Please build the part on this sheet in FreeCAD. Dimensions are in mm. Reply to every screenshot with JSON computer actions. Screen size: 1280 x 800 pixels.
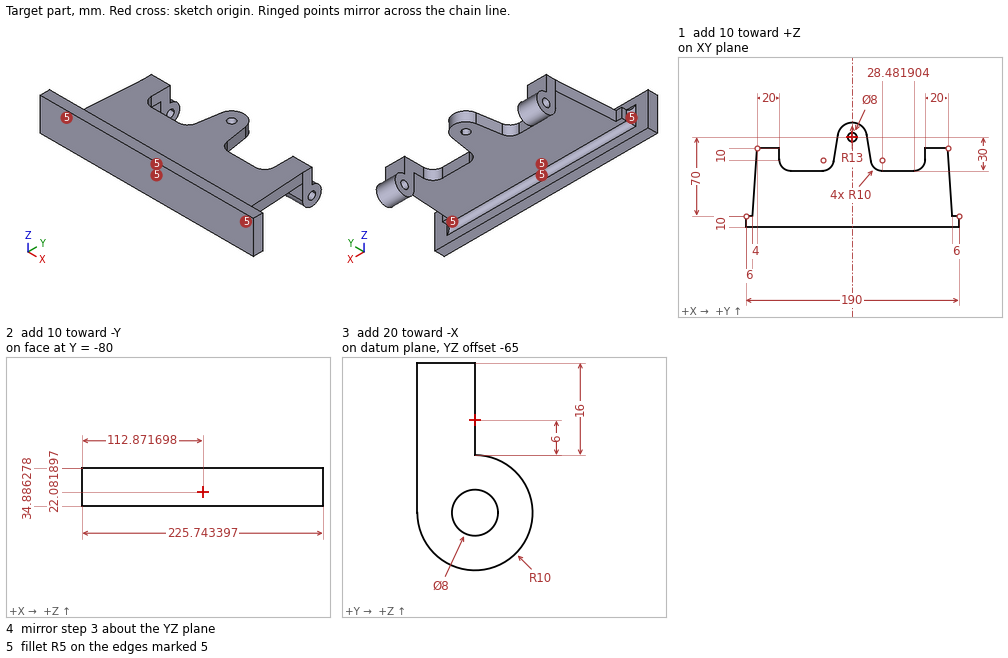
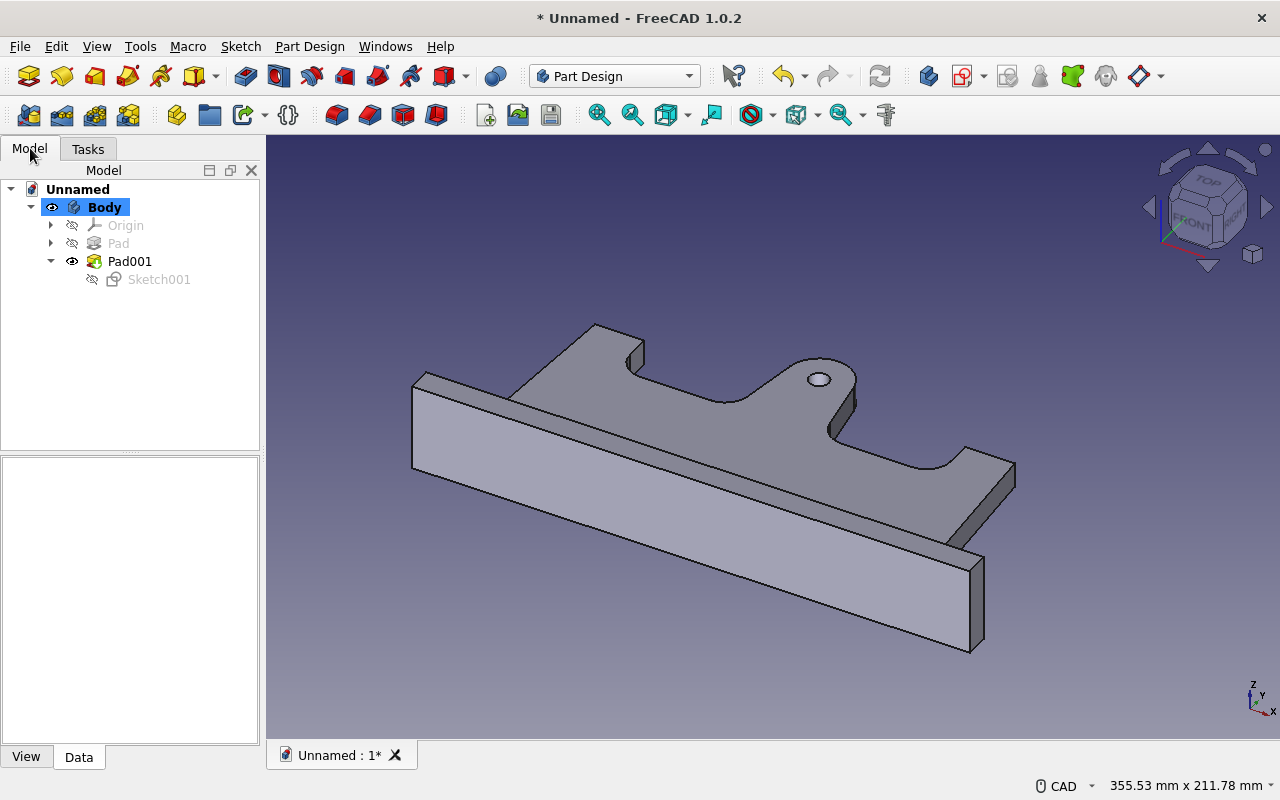
{"action": "left_click", "coordinate": [51, 225]}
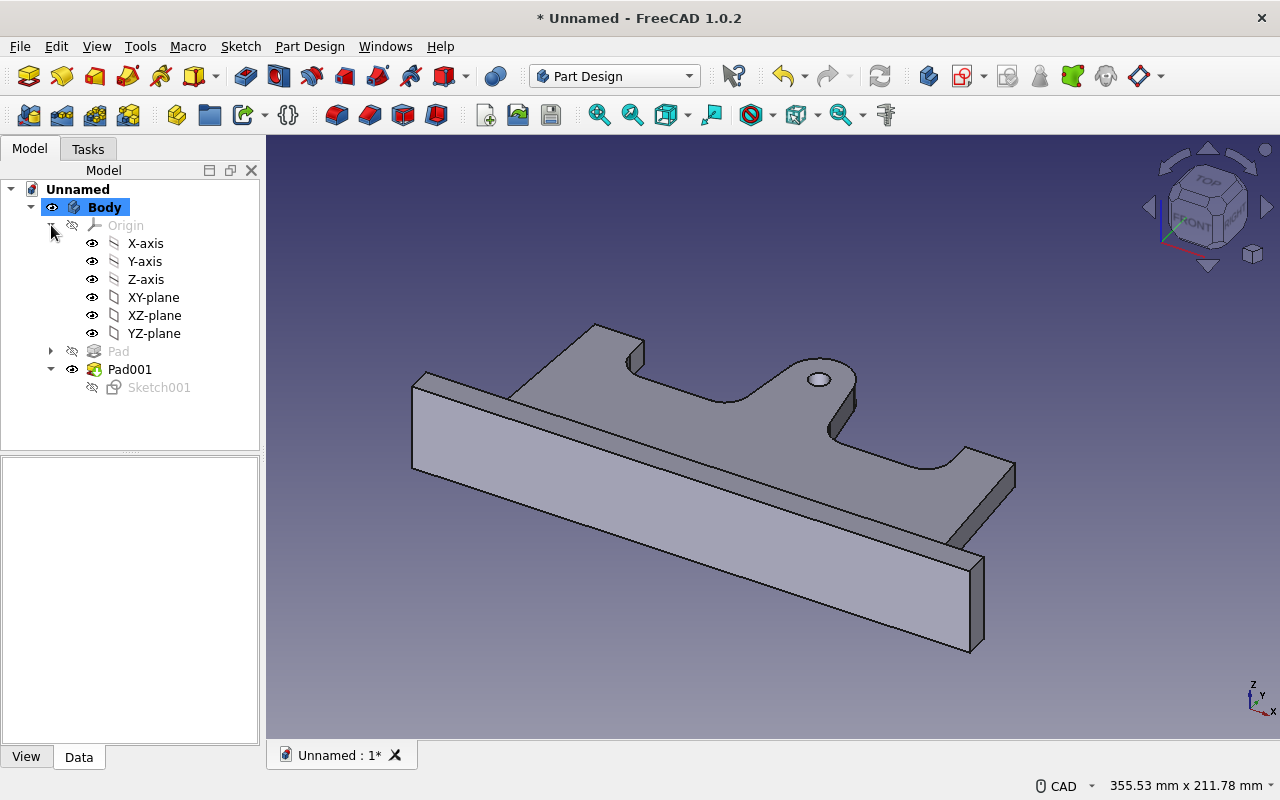
{"action": "left_click", "coordinate": [137, 333]}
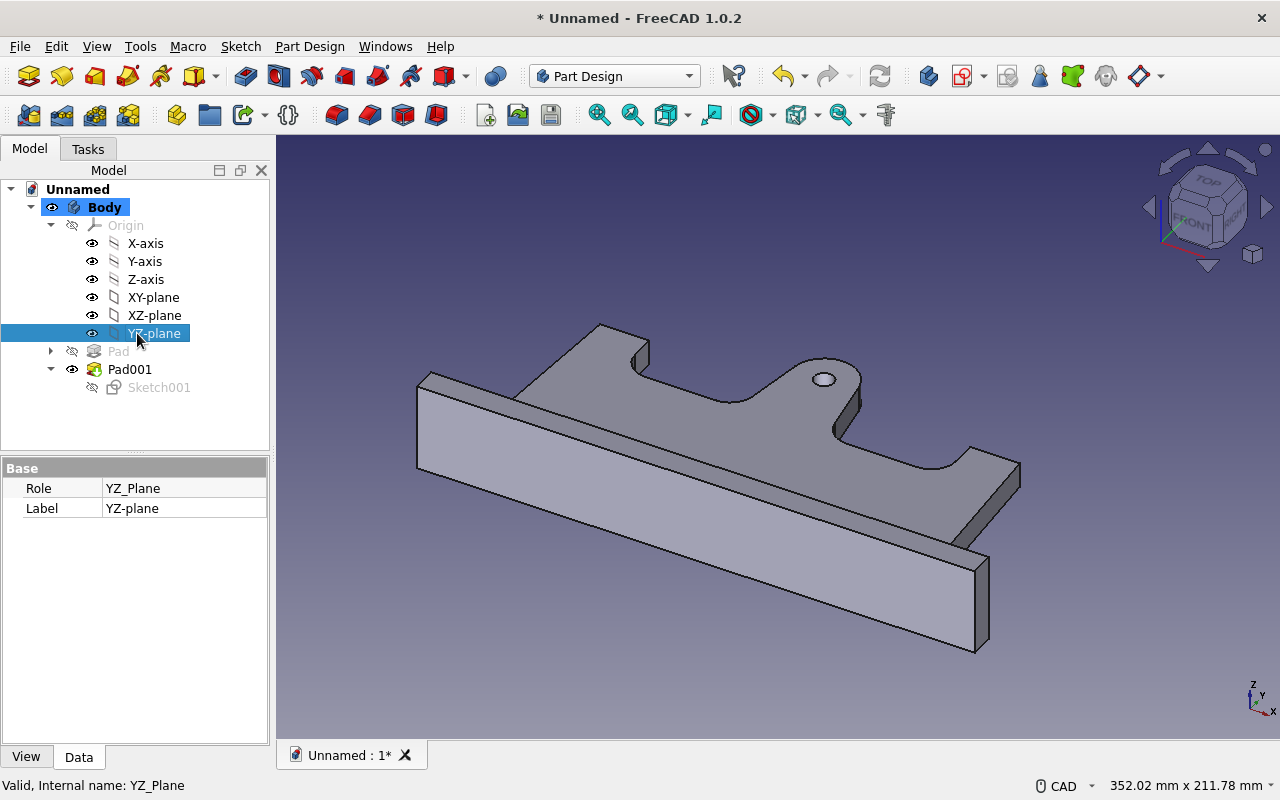
{"action": "left_click", "coordinate": [1138, 76]}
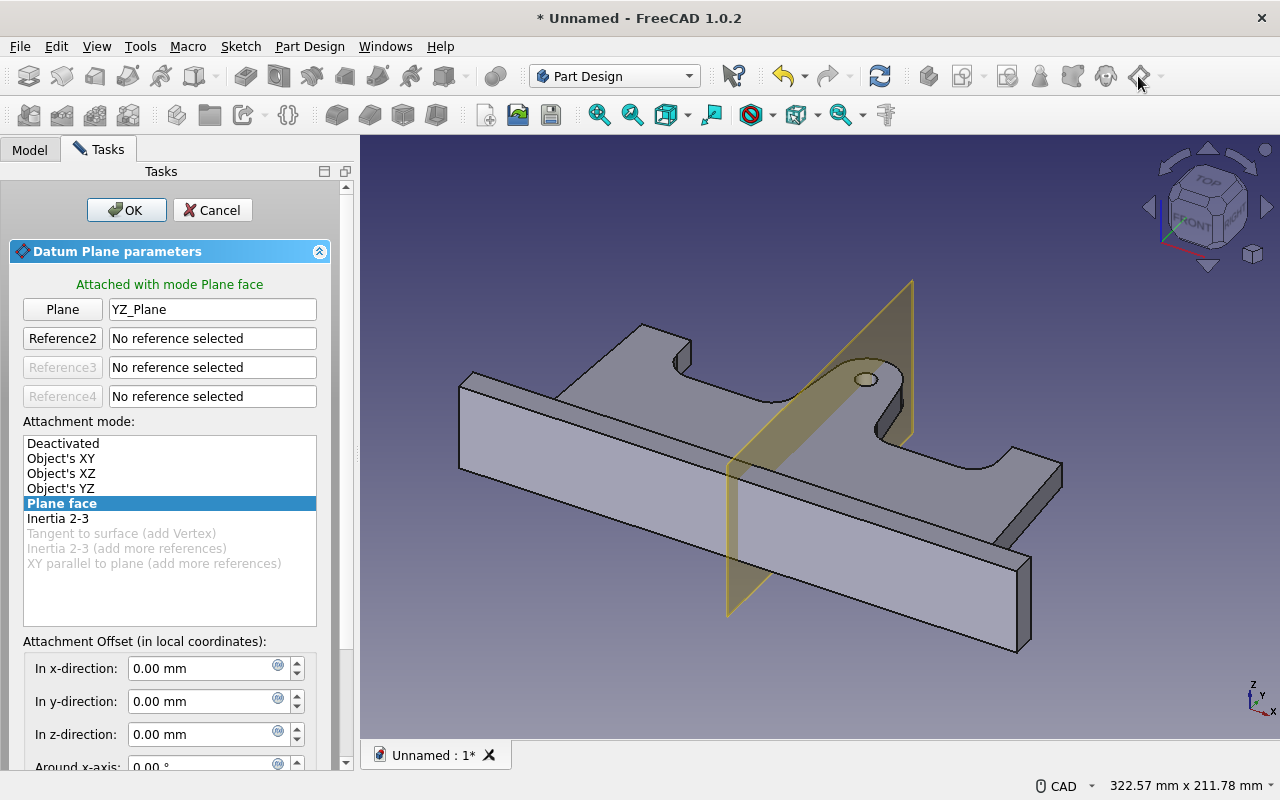
{"action": "triple_click", "coordinate": [210, 734]}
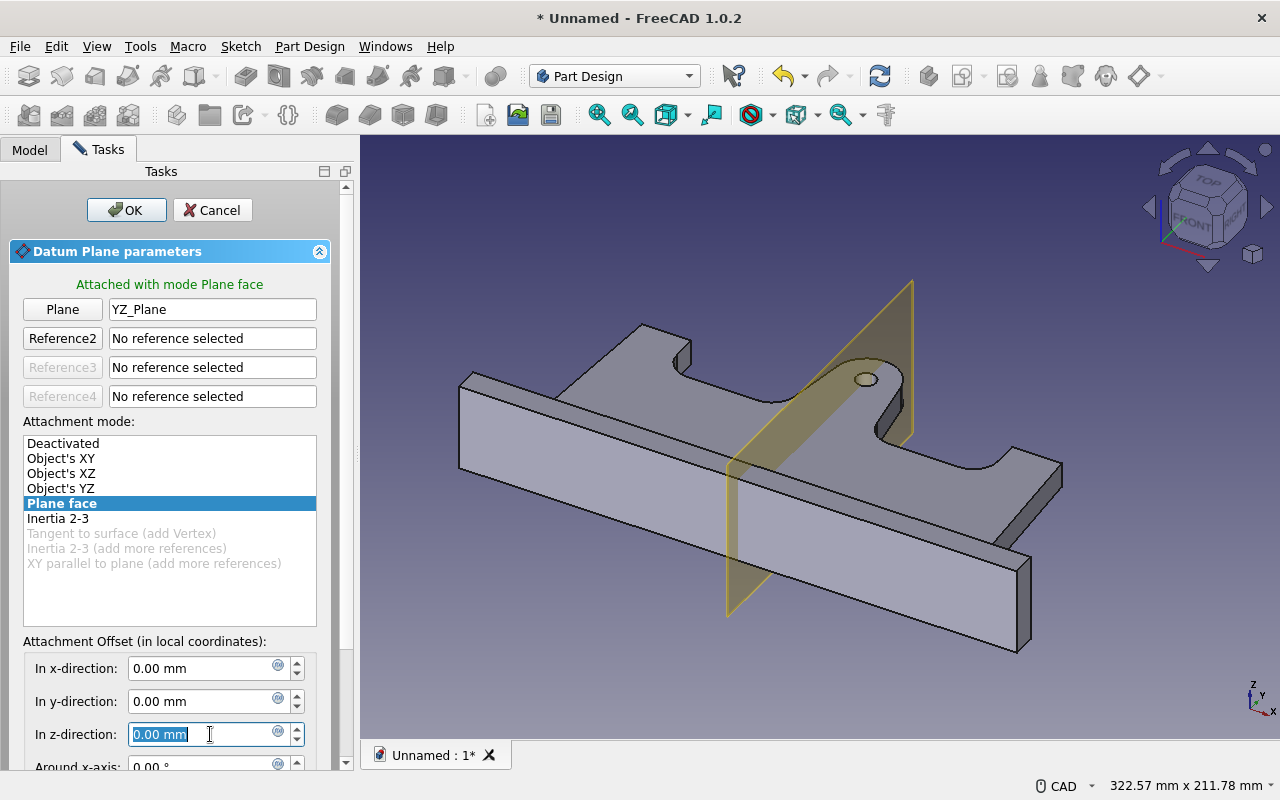
{"action": "type", "text": "-65"}
{"action": "key", "text": "Tab"}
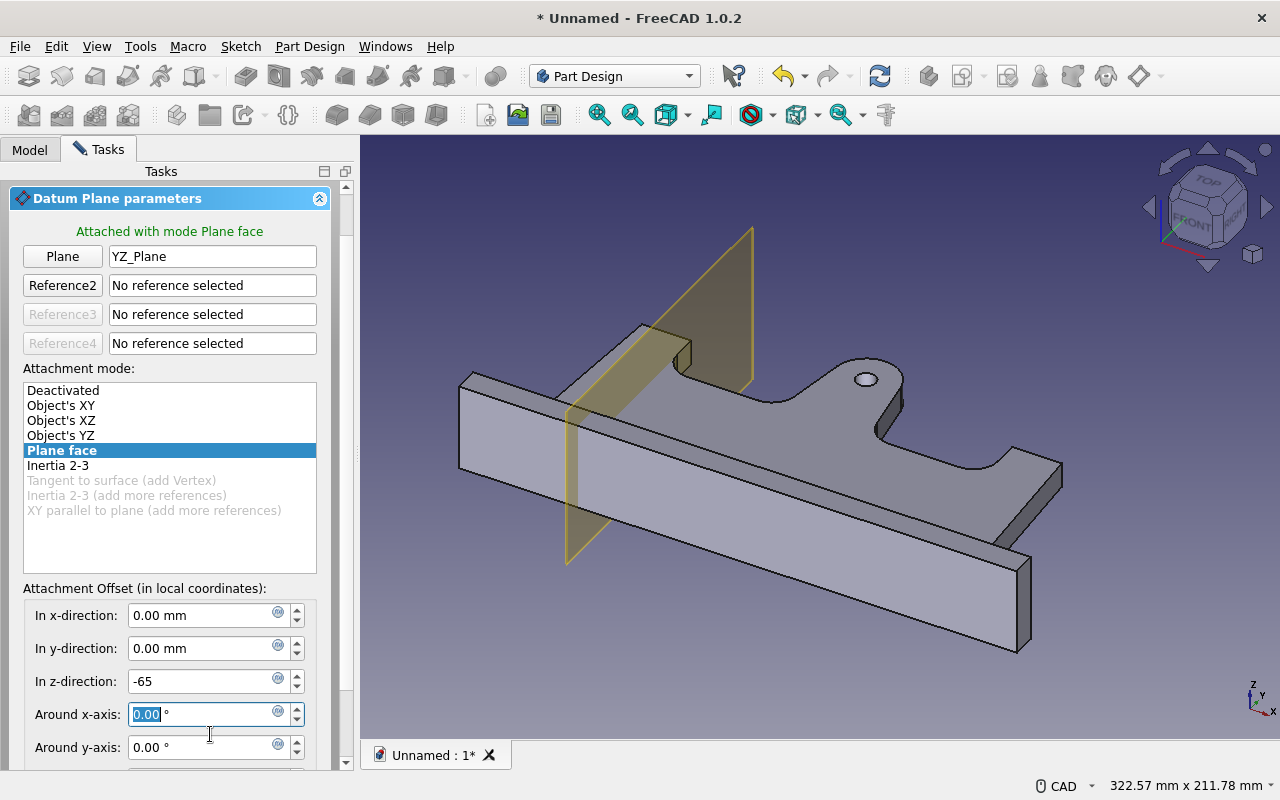
{"action": "scroll", "coordinate": [346, 476], "scroll_direction": "up", "scroll_amount": 2}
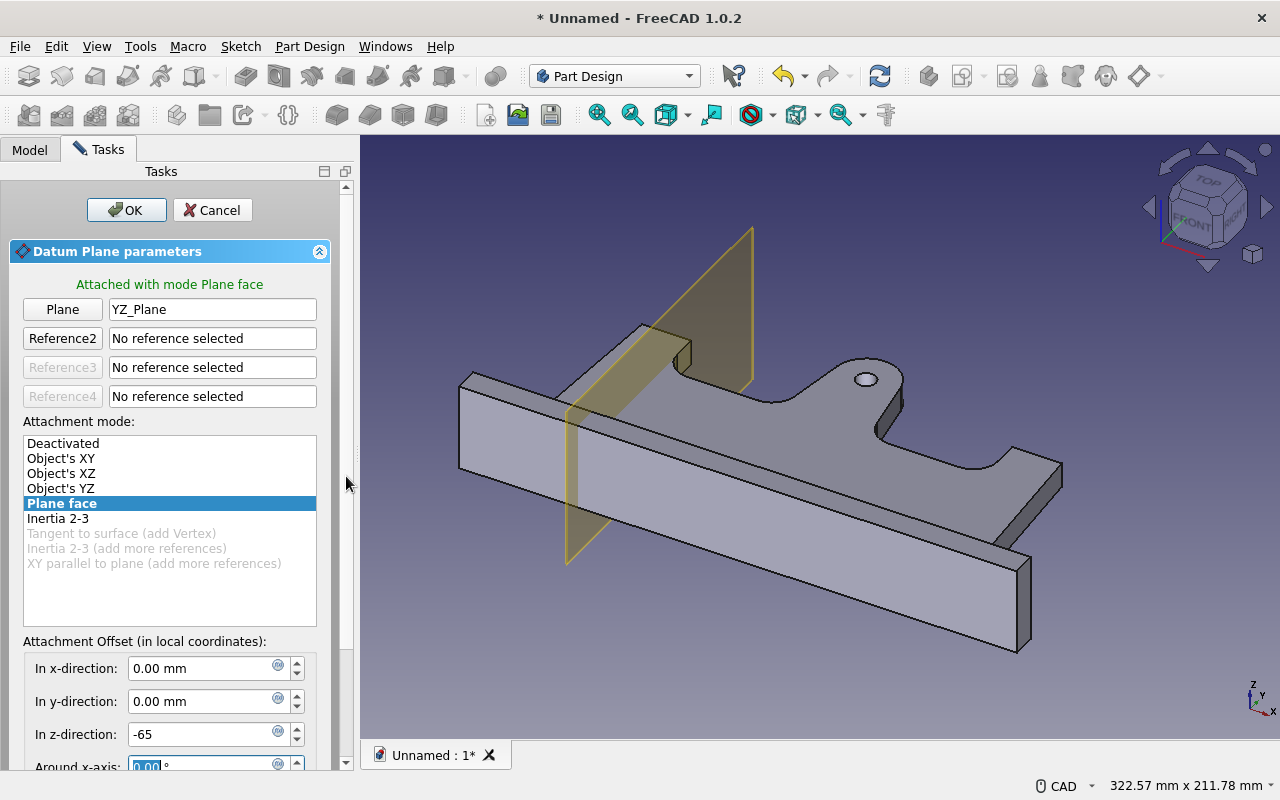
{"action": "left_click", "coordinate": [127, 210]}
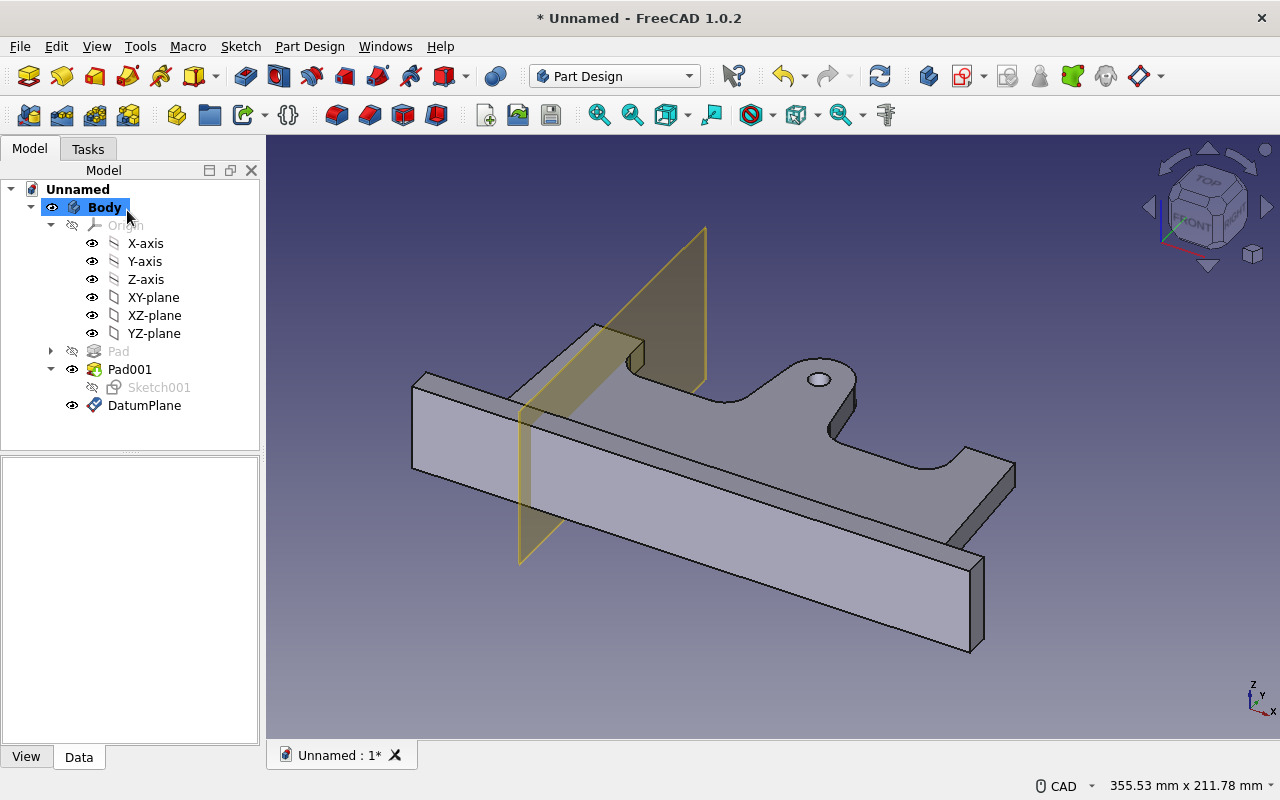
{"action": "left_click", "coordinate": [117, 405]}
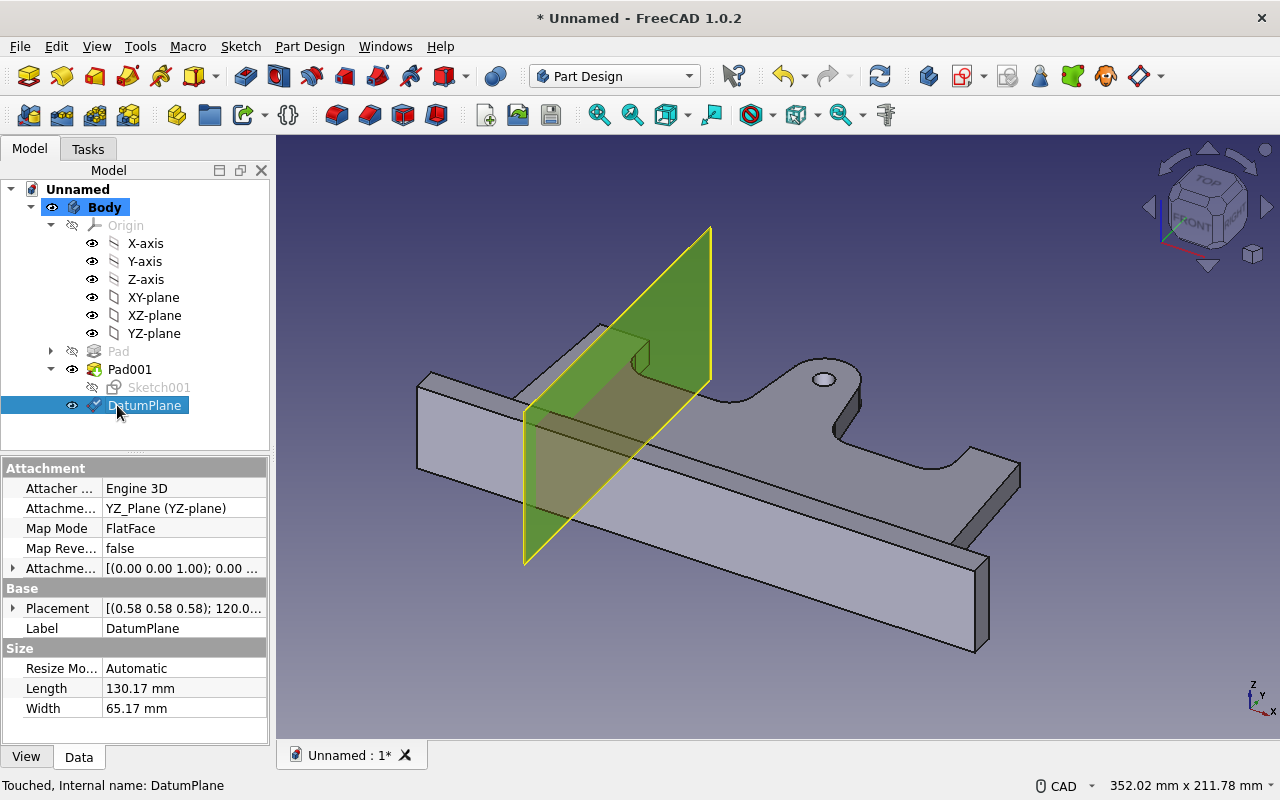
{"action": "left_click", "coordinate": [962, 76]}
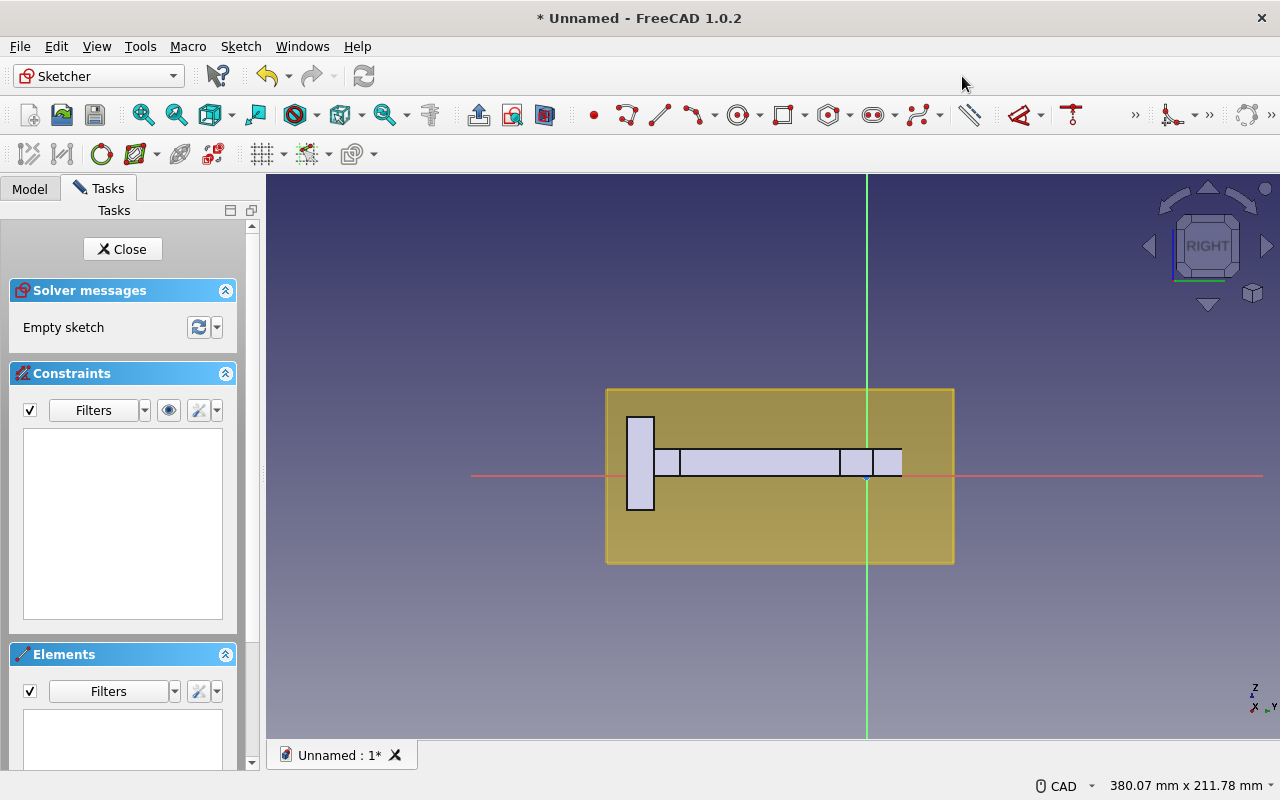
{"action": "left_click", "coordinate": [545, 116]}